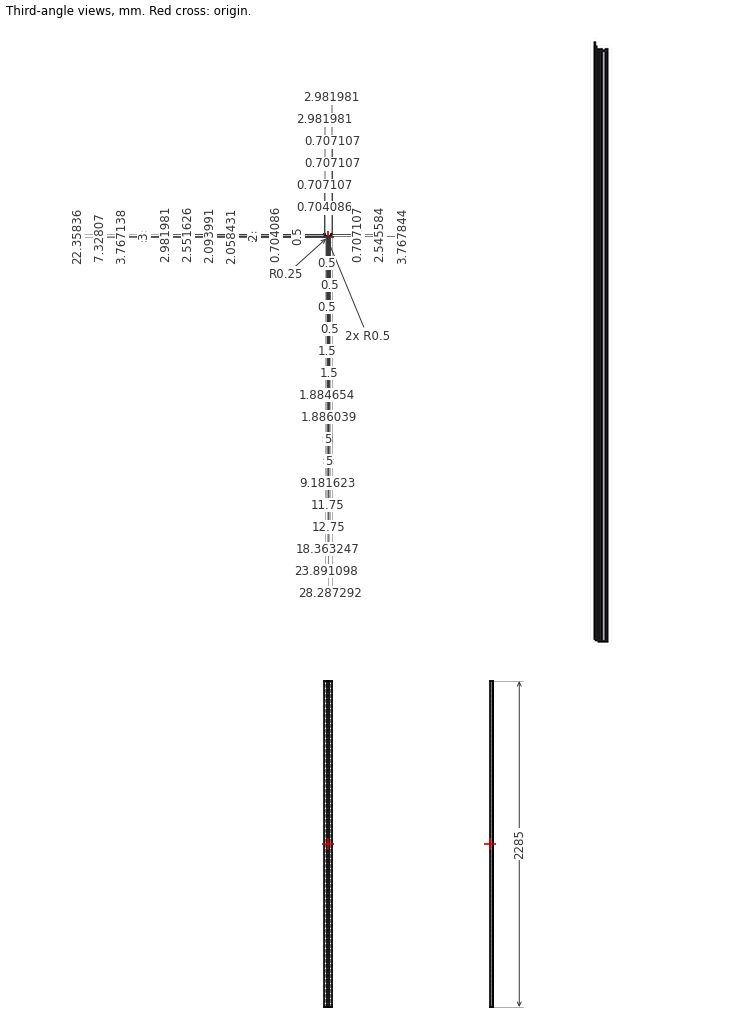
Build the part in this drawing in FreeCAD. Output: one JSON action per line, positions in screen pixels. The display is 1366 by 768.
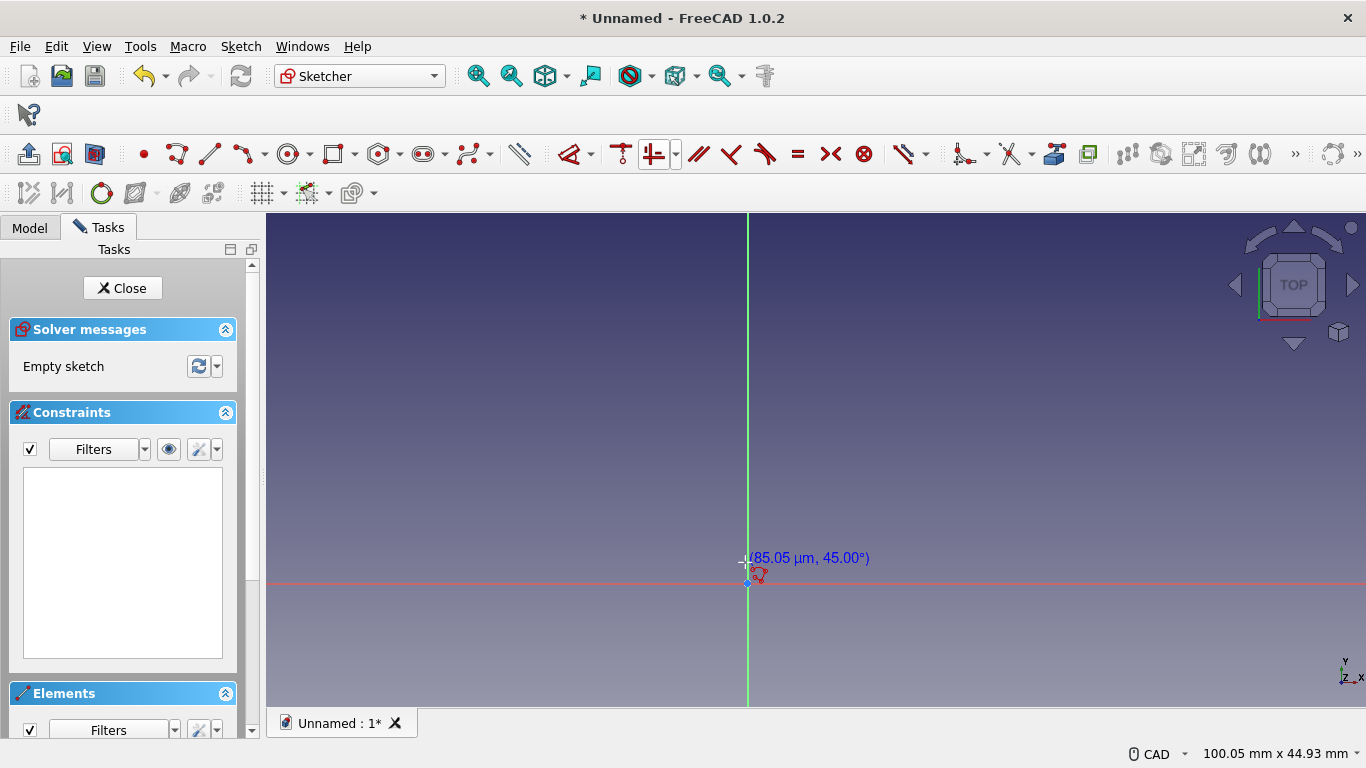
{"action": "left_click", "coordinate": [690, 562]}
{"action": "left_click", "coordinate": [690, 529]}
{"action": "left_click", "coordinate": [673, 529]}
{"action": "left_click", "coordinate": [673, 562]}
{"action": "left_click", "coordinate": [653, 562]}
{"action": "left_click", "coordinate": [618, 528]}
{"action": "left_click", "coordinate": [618, 486]}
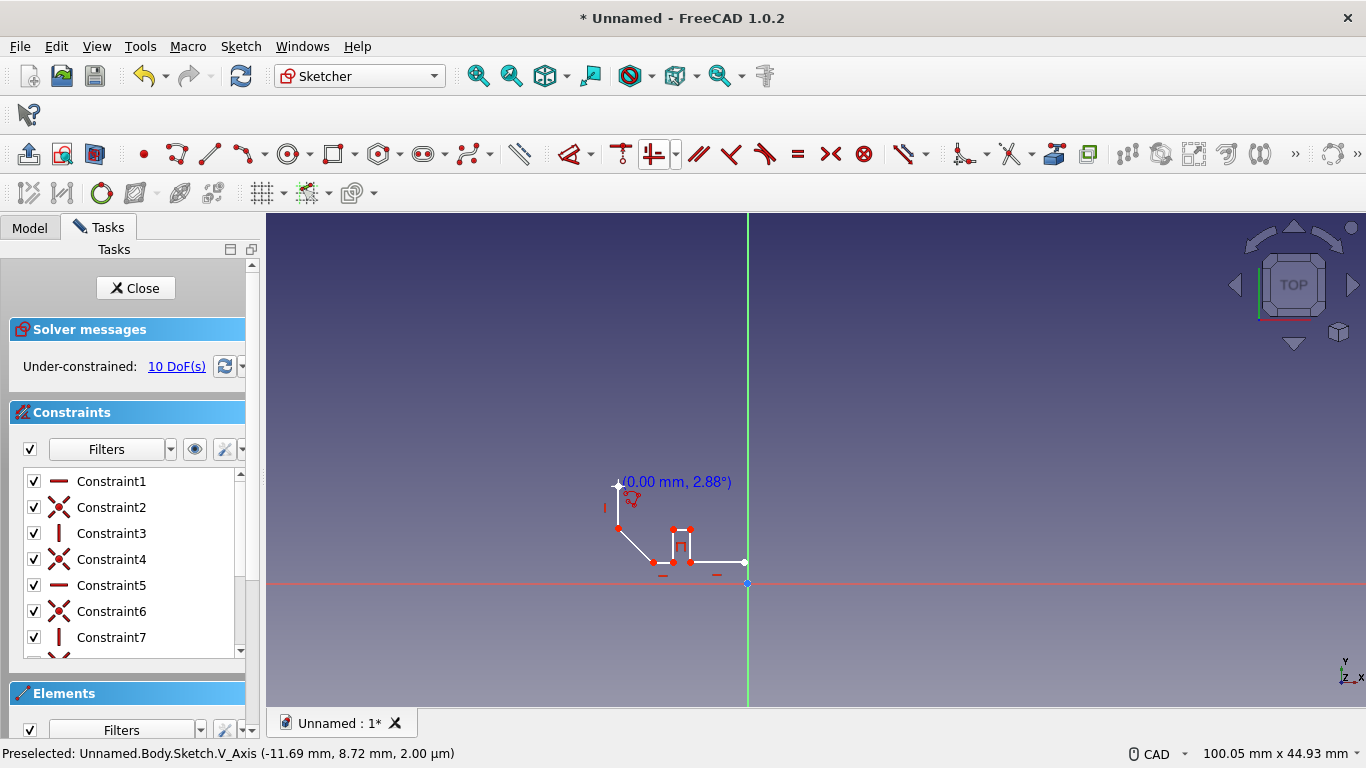
{"action": "scroll", "coordinate": [613, 481], "scroll_direction": "up", "scroll_amount": 4}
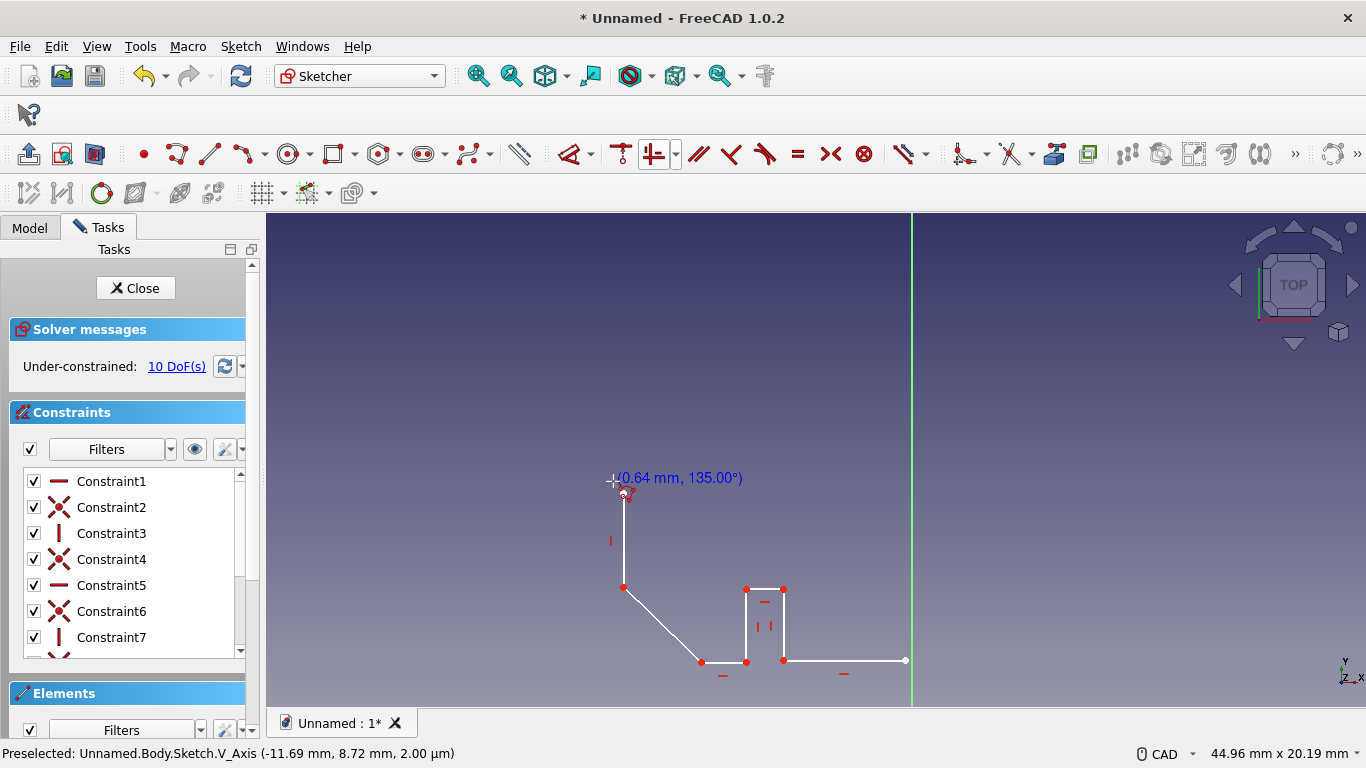
{"action": "left_click", "coordinate": [612, 480]}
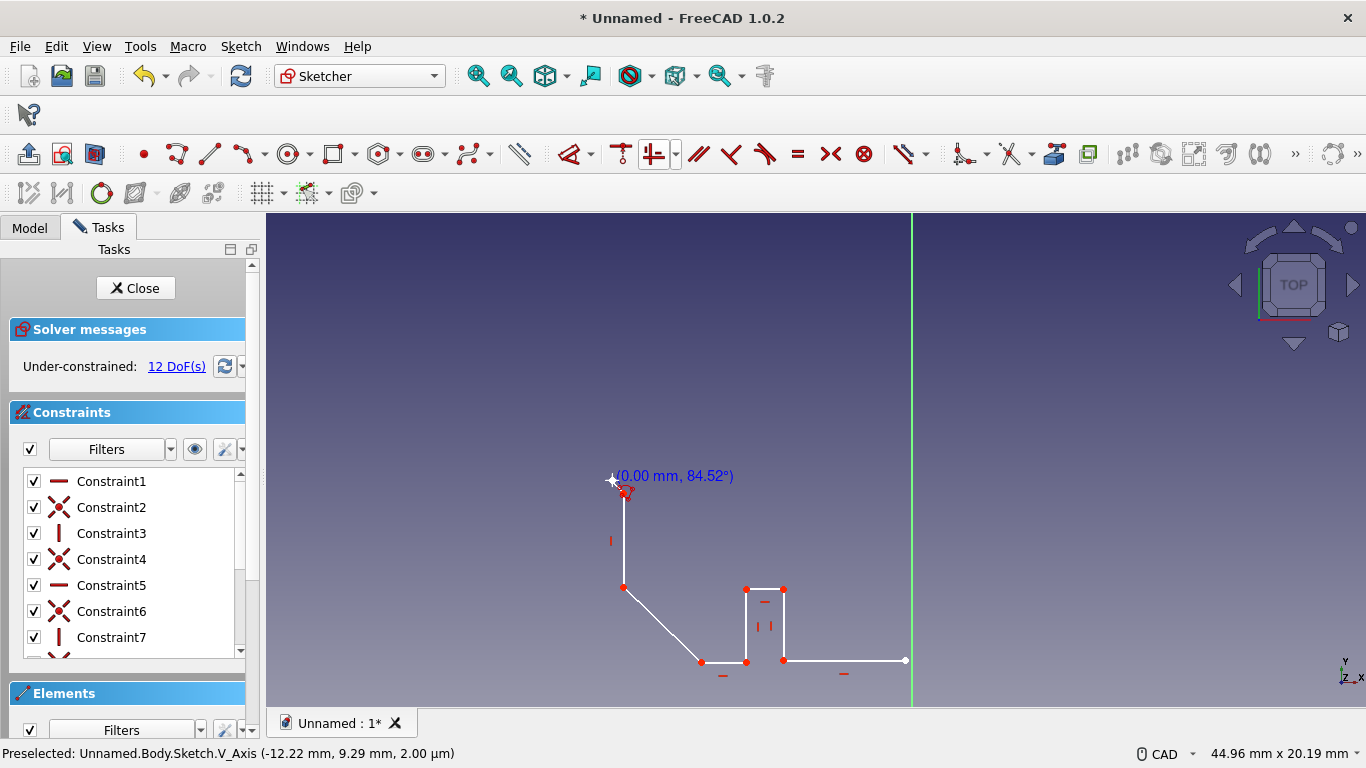
{"action": "scroll", "coordinate": [600, 480], "scroll_direction": "up", "scroll_amount": 2}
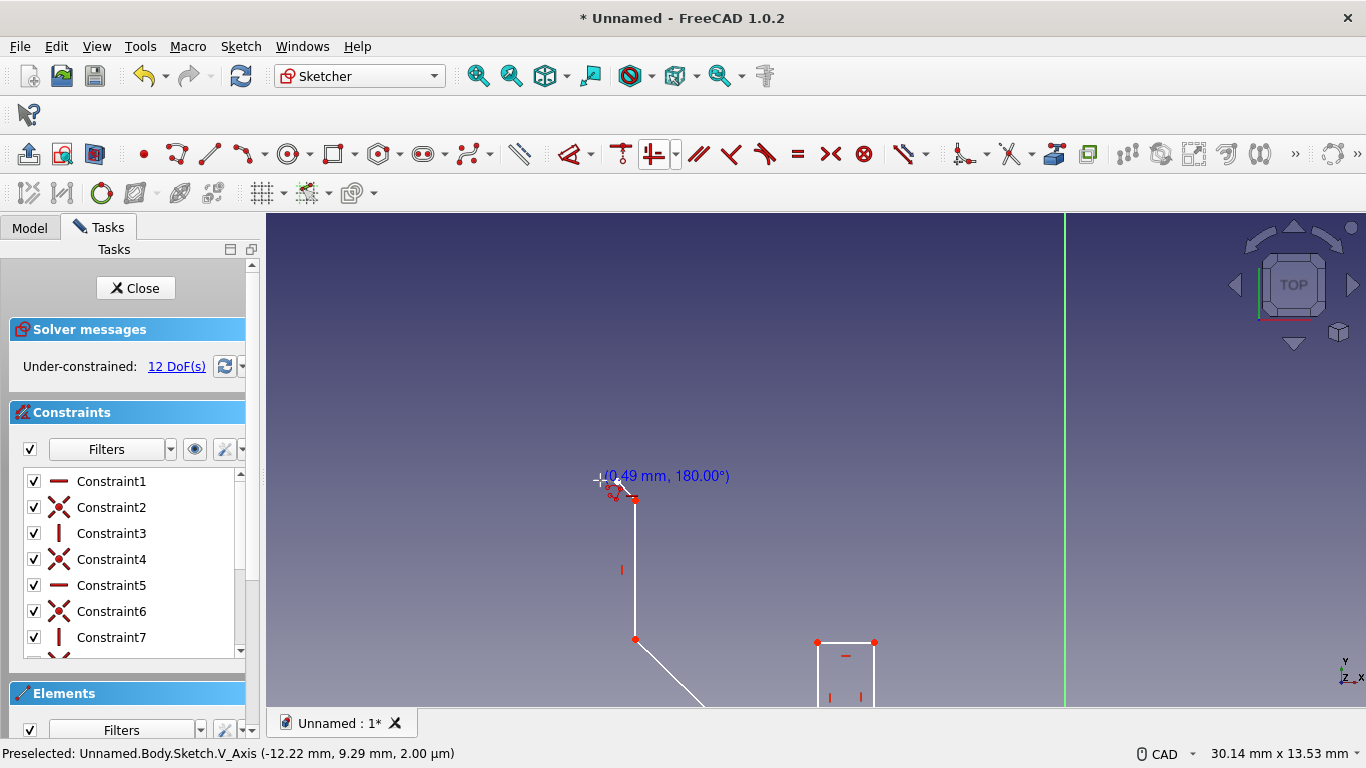
{"action": "left_click", "coordinate": [600, 480]}
{"action": "left_click", "coordinate": [600, 554]}
{"action": "right_click", "coordinate": [600, 554]}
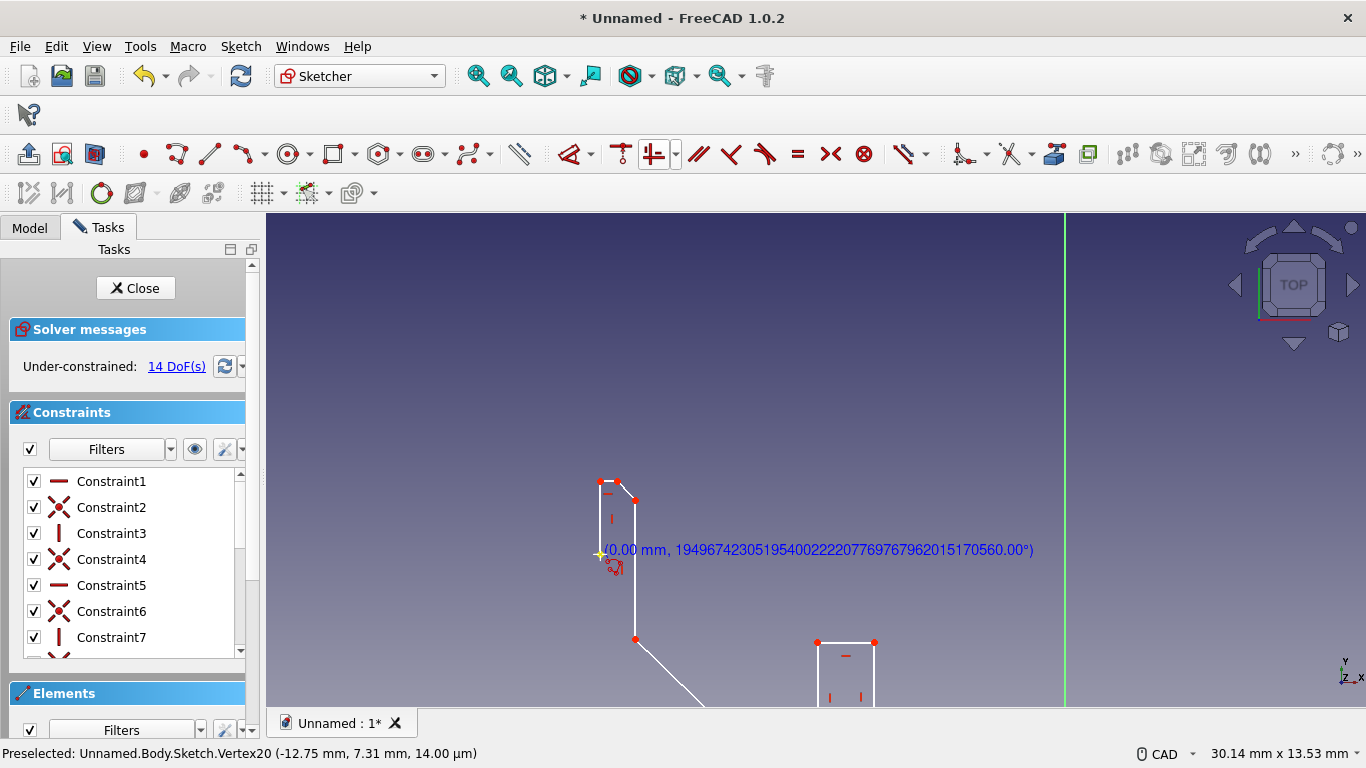
{"action": "left_click", "coordinate": [569, 567]}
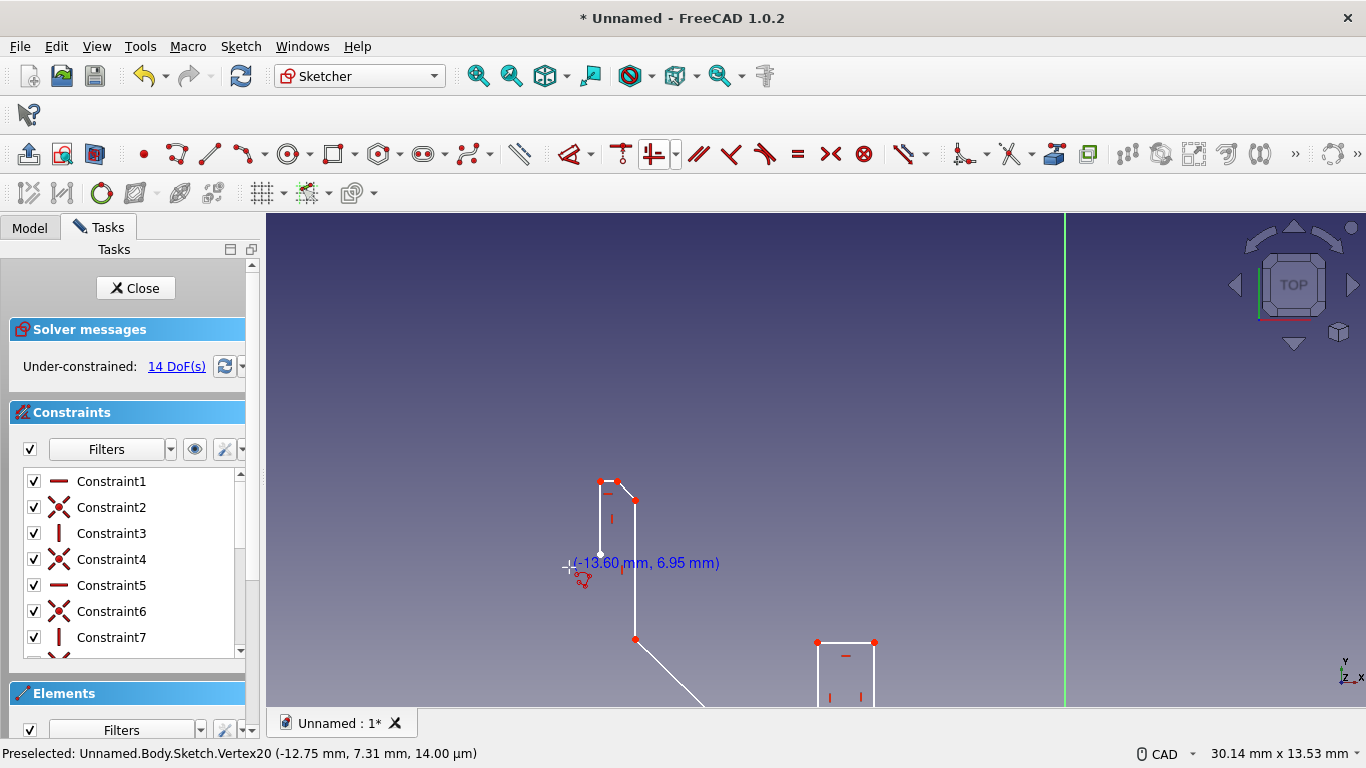
{"action": "scroll", "coordinate": [610, 480], "scroll_direction": "down", "scroll_amount": 6}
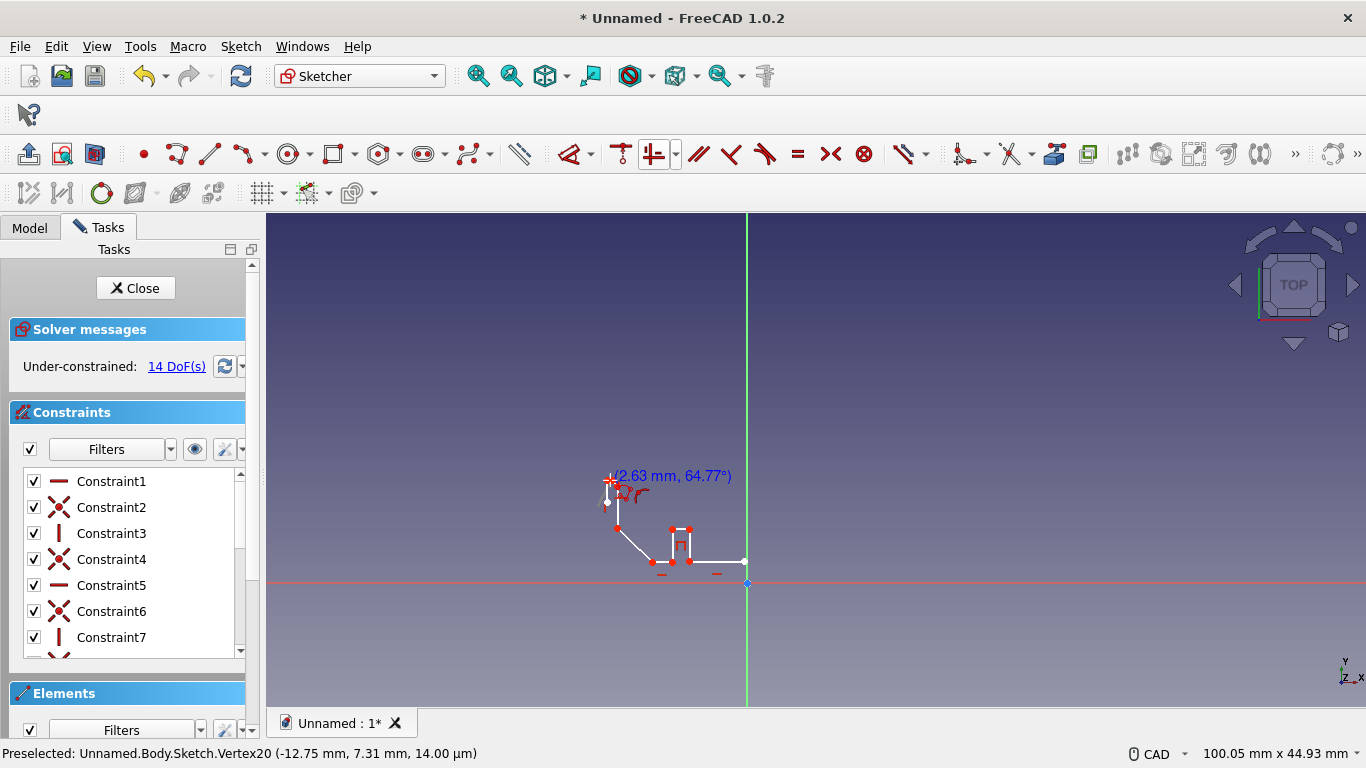
{"action": "left_click", "coordinate": [485, 393]}
{"action": "left_click", "coordinate": [485, 370]}
{"action": "left_click", "coordinate": [452, 337]}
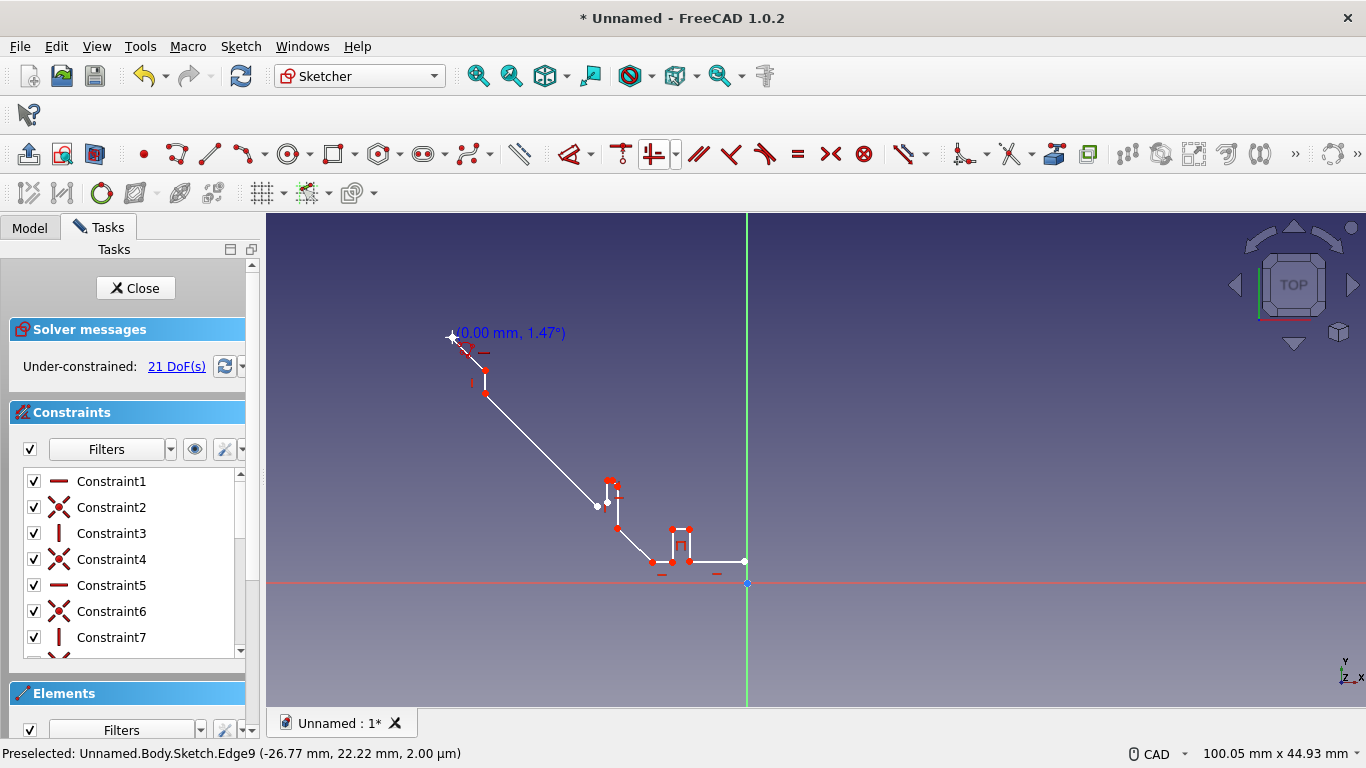
{"action": "scroll", "coordinate": [444, 337], "scroll_direction": "up", "scroll_amount": 4}